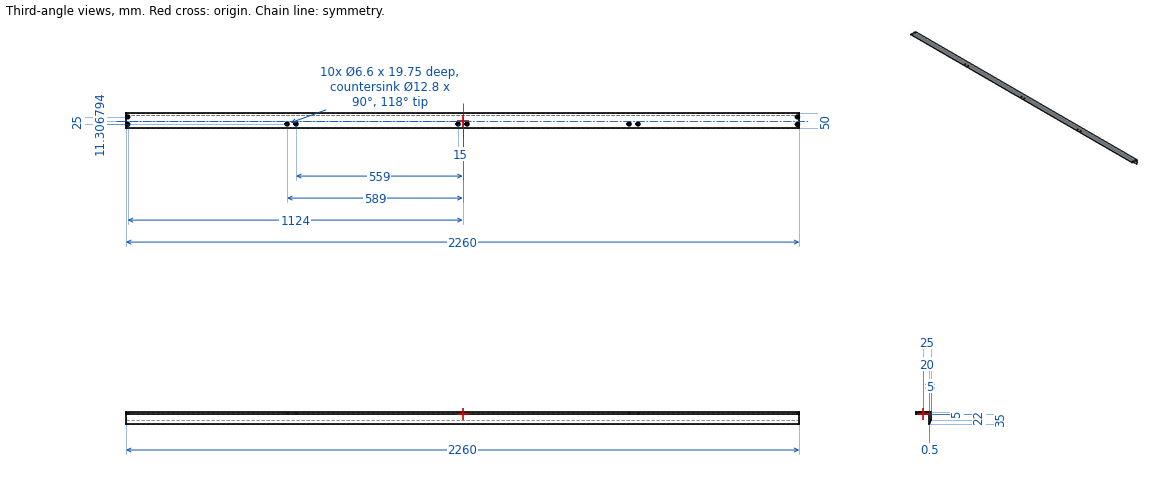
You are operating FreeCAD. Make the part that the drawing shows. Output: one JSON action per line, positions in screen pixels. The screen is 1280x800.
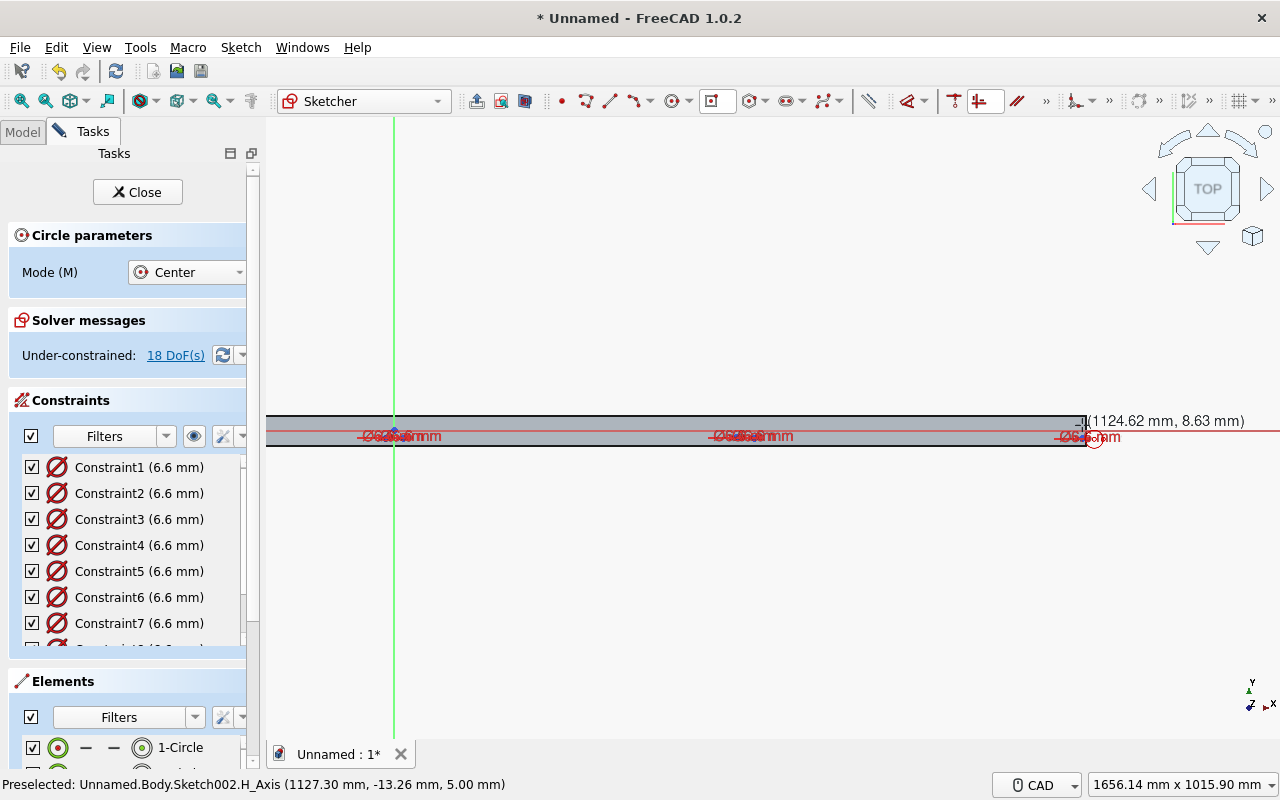
{"action": "scroll", "coordinate": [1083, 424], "scroll_direction": "up", "scroll_amount": 7}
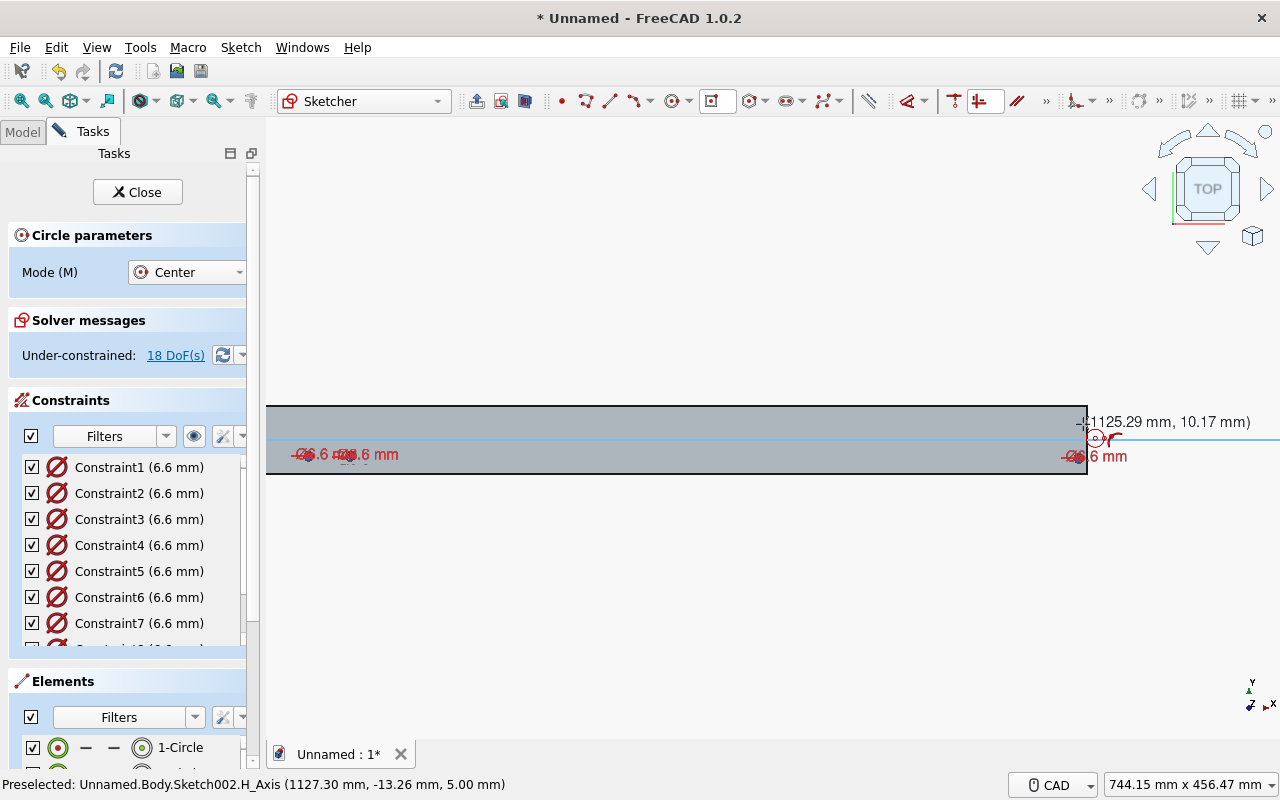
{"action": "left_click", "coordinate": [1079, 423]}
{"action": "mouse_move", "coordinate": [1082, 420]}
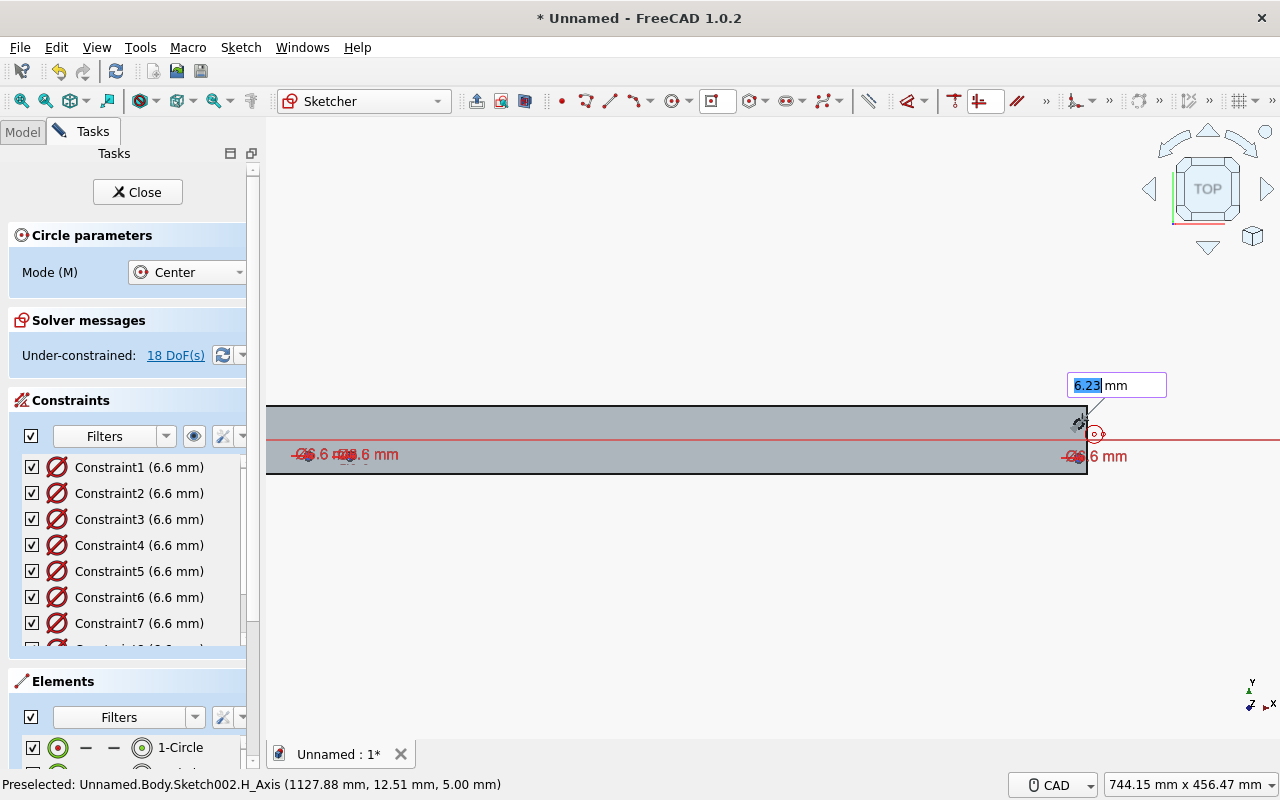
{"action": "type", "text": "6.6"}
{"action": "key", "text": "Return"}
{"action": "key", "text": "Escape"}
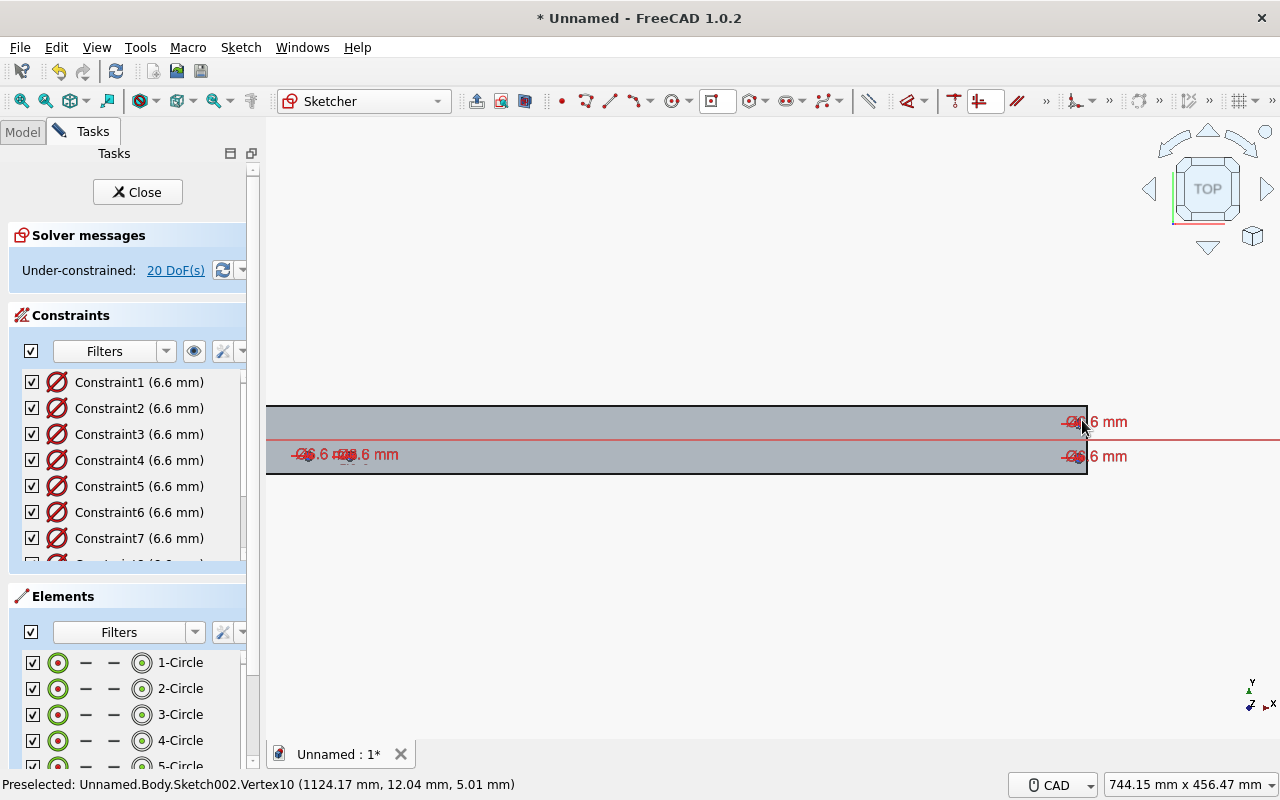
{"action": "scroll", "coordinate": [997, 425], "scroll_direction": "down", "scroll_amount": 8}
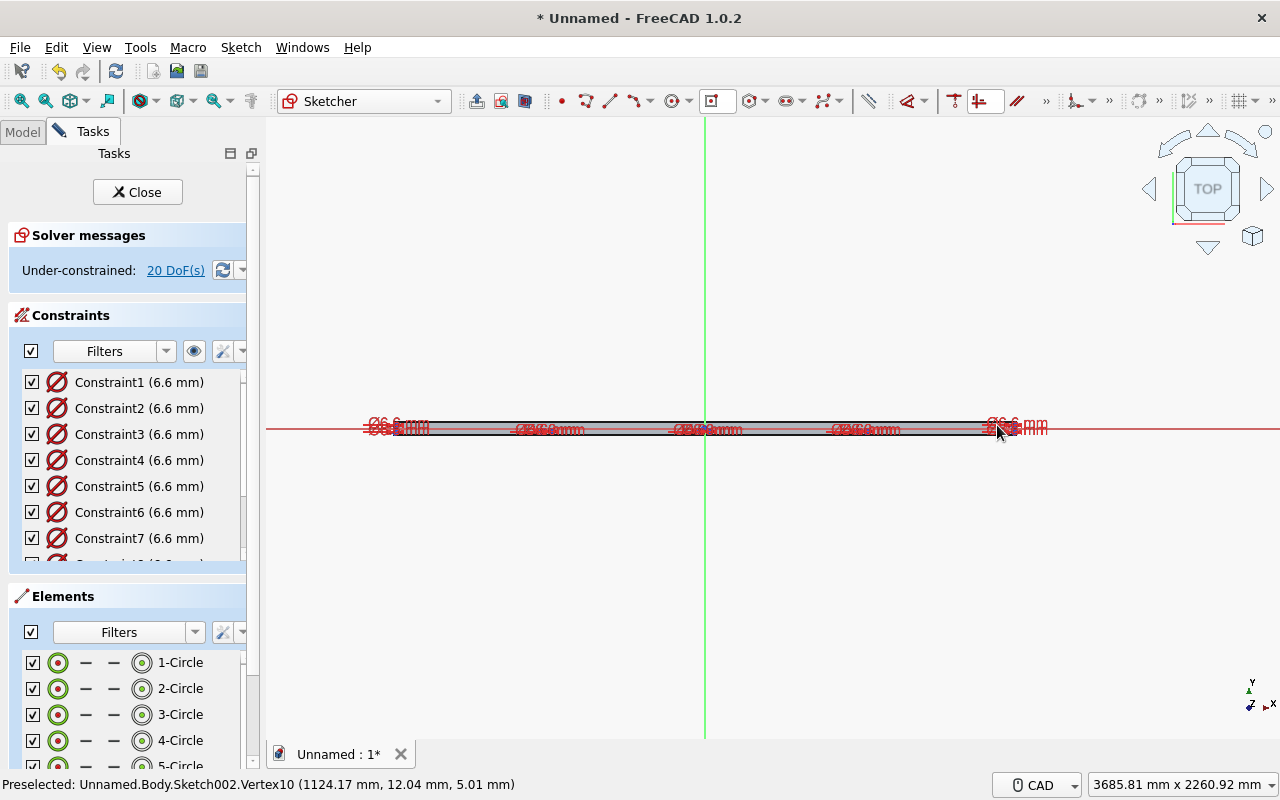
{"action": "scroll", "coordinate": [701, 432], "scroll_direction": "up", "scroll_amount": 5}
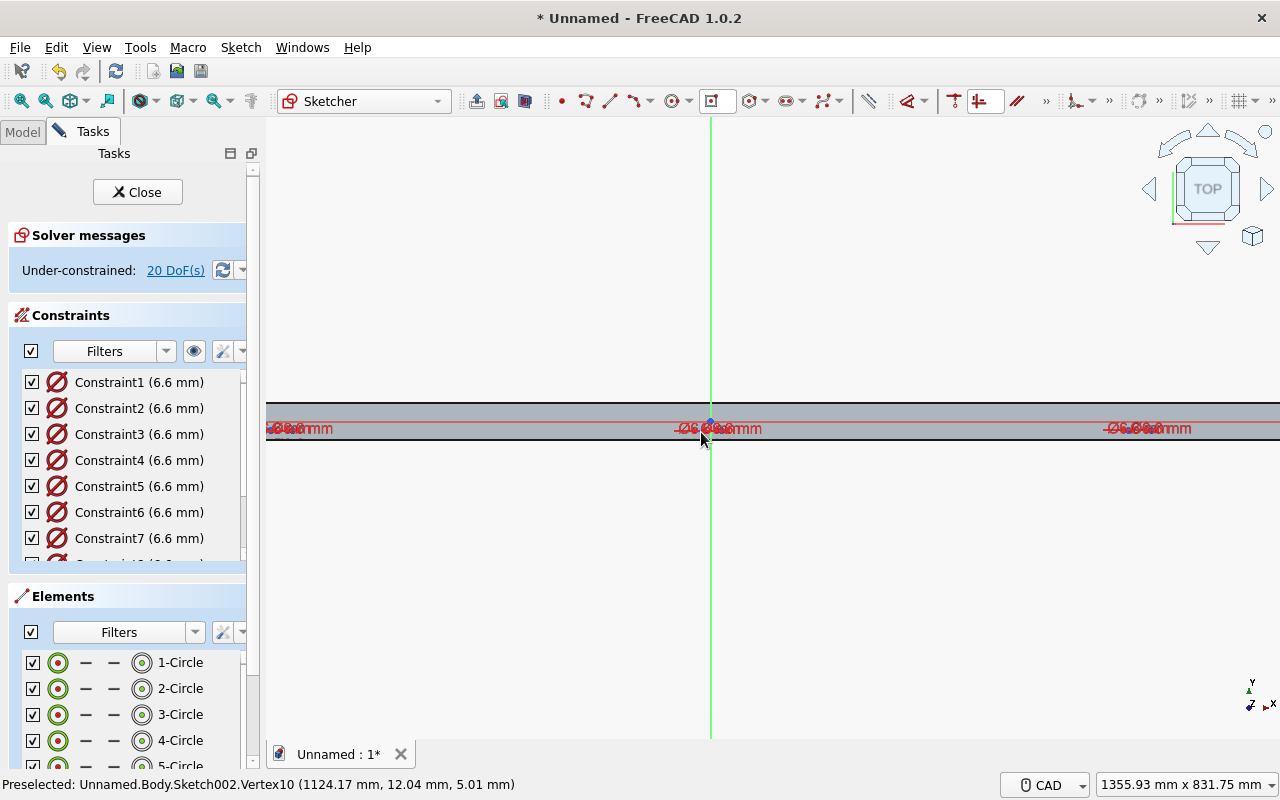
{"action": "left_click", "coordinate": [700, 431]}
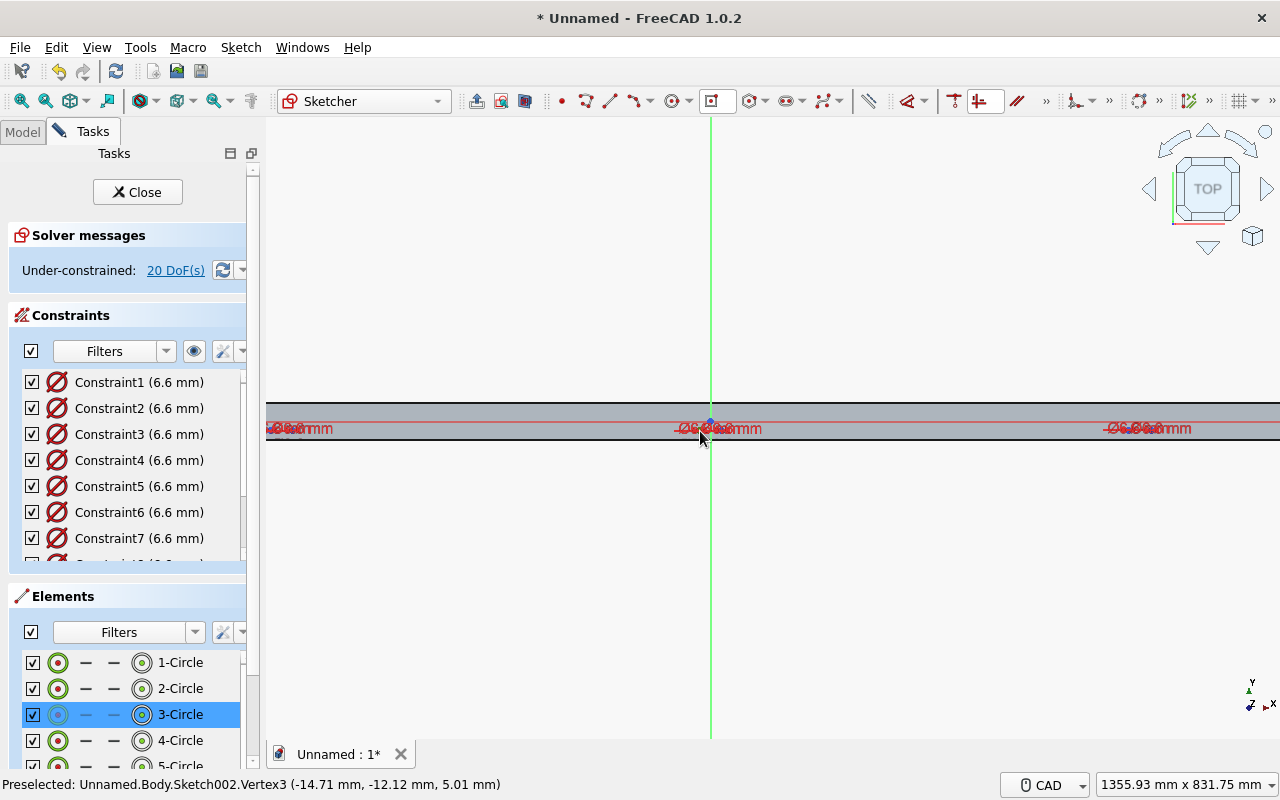
{"action": "left_click", "coordinate": [722, 431]}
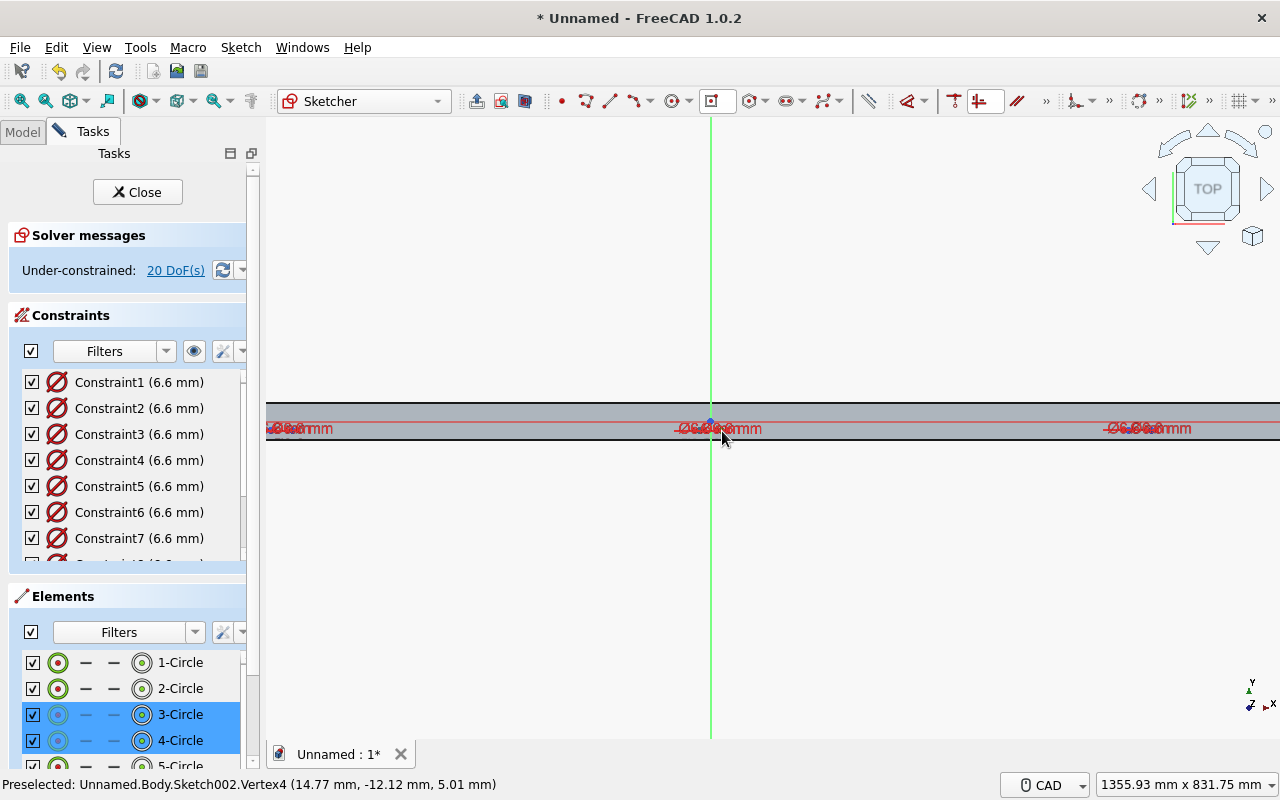
{"action": "left_click", "coordinate": [711, 671]}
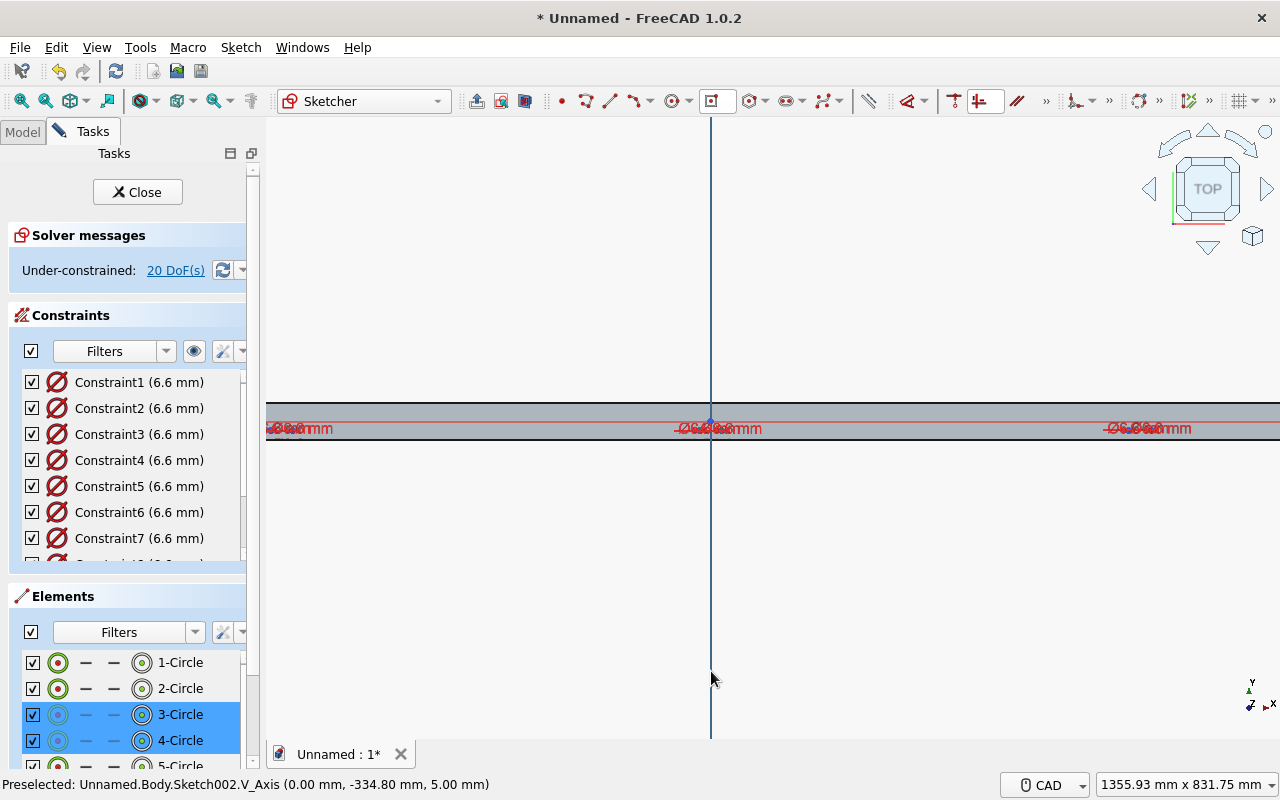
{"action": "key", "text": "s"}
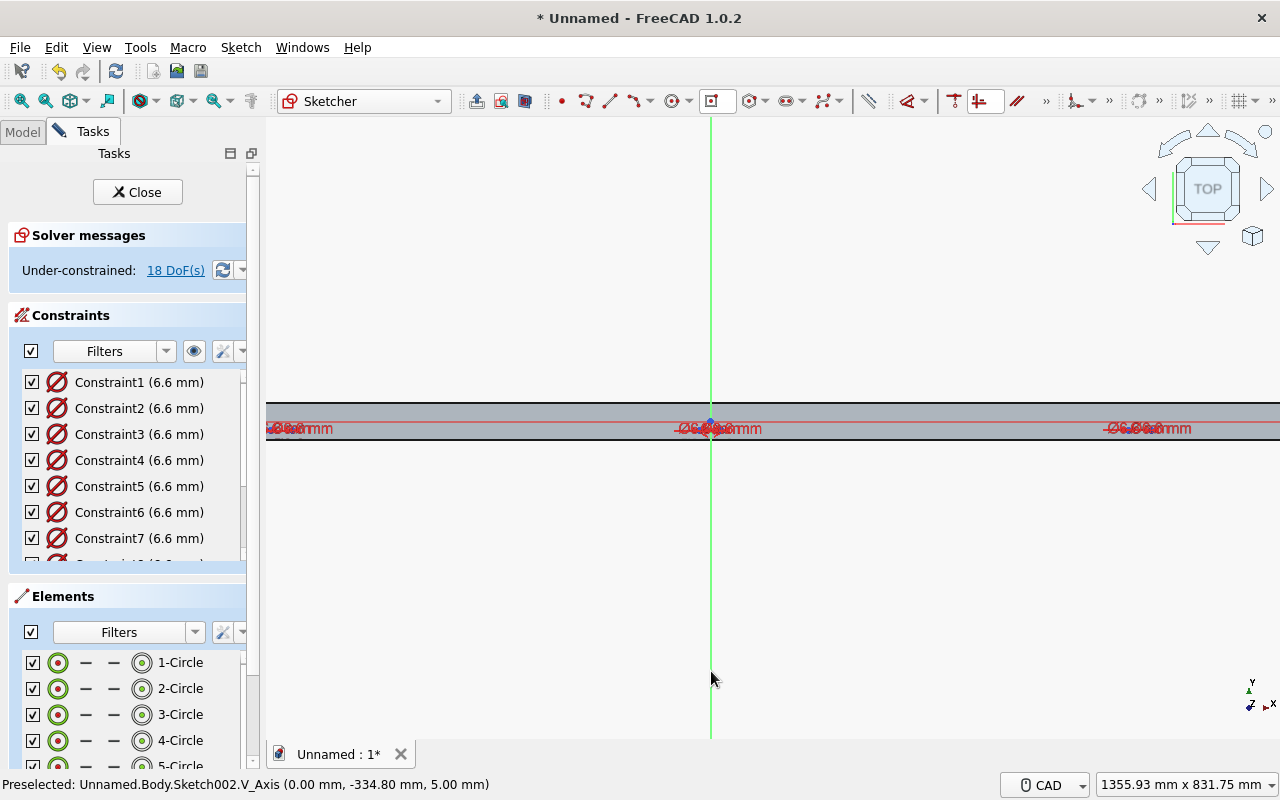
{"action": "scroll", "coordinate": [701, 432], "scroll_direction": "down", "scroll_amount": 5}